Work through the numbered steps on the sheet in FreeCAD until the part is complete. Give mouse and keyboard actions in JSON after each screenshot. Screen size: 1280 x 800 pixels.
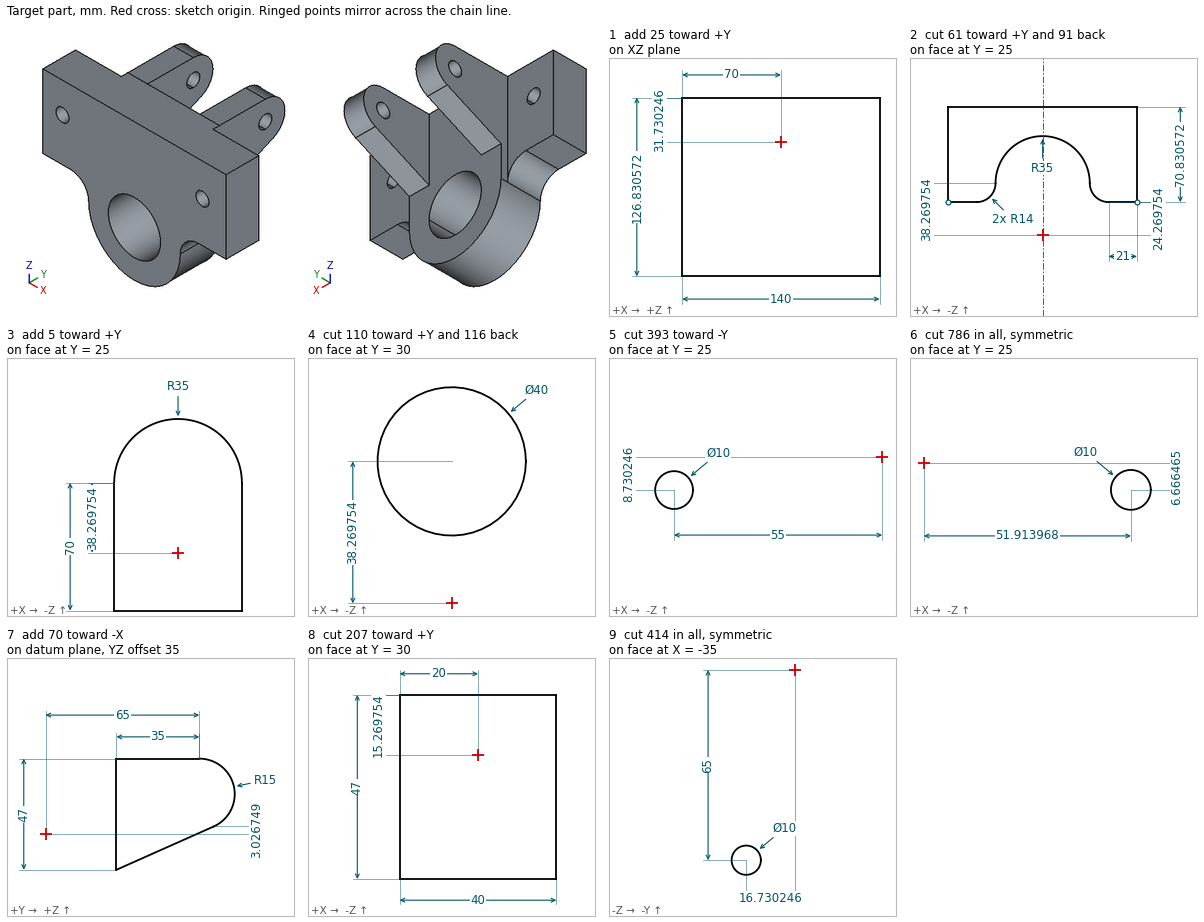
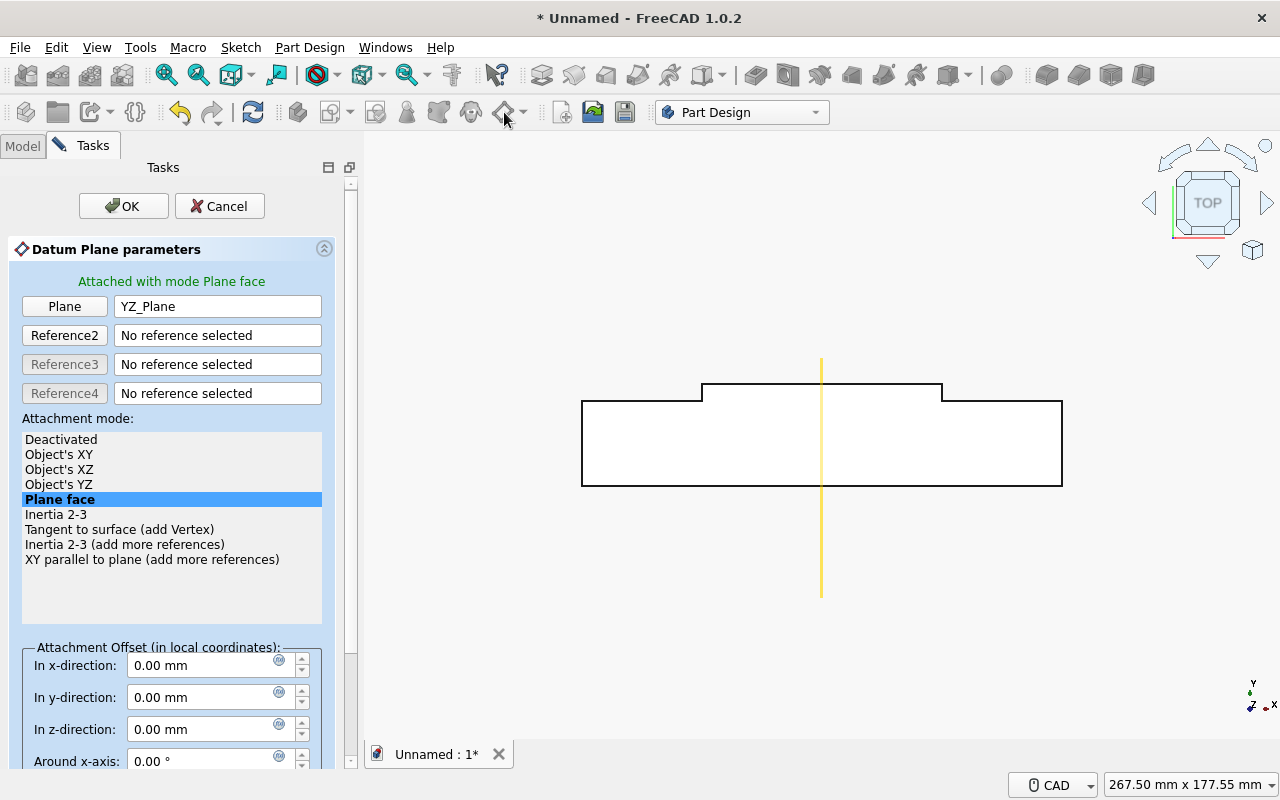
{"action": "triple_click", "coordinate": [210, 729]}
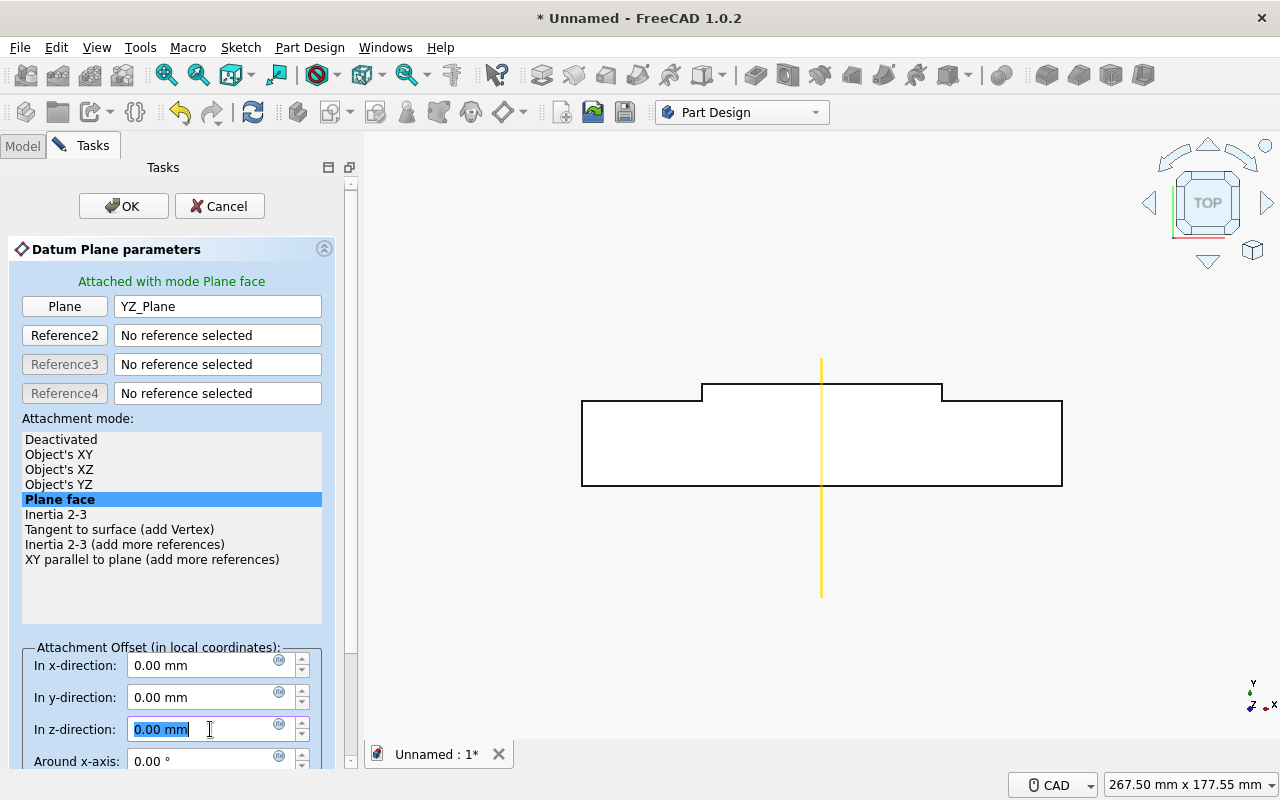
{"action": "type", "text": "35"}
{"action": "key", "text": "Tab"}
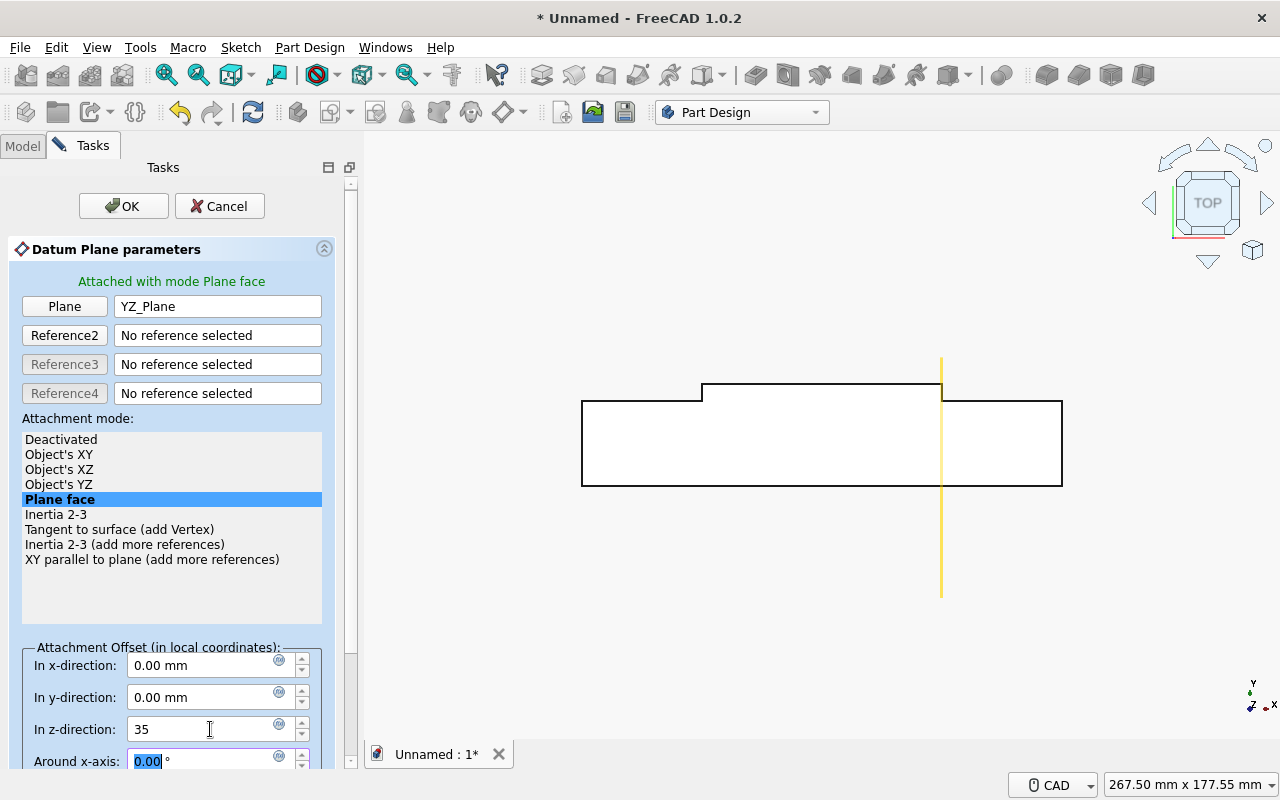
{"action": "left_click", "coordinate": [124, 206]}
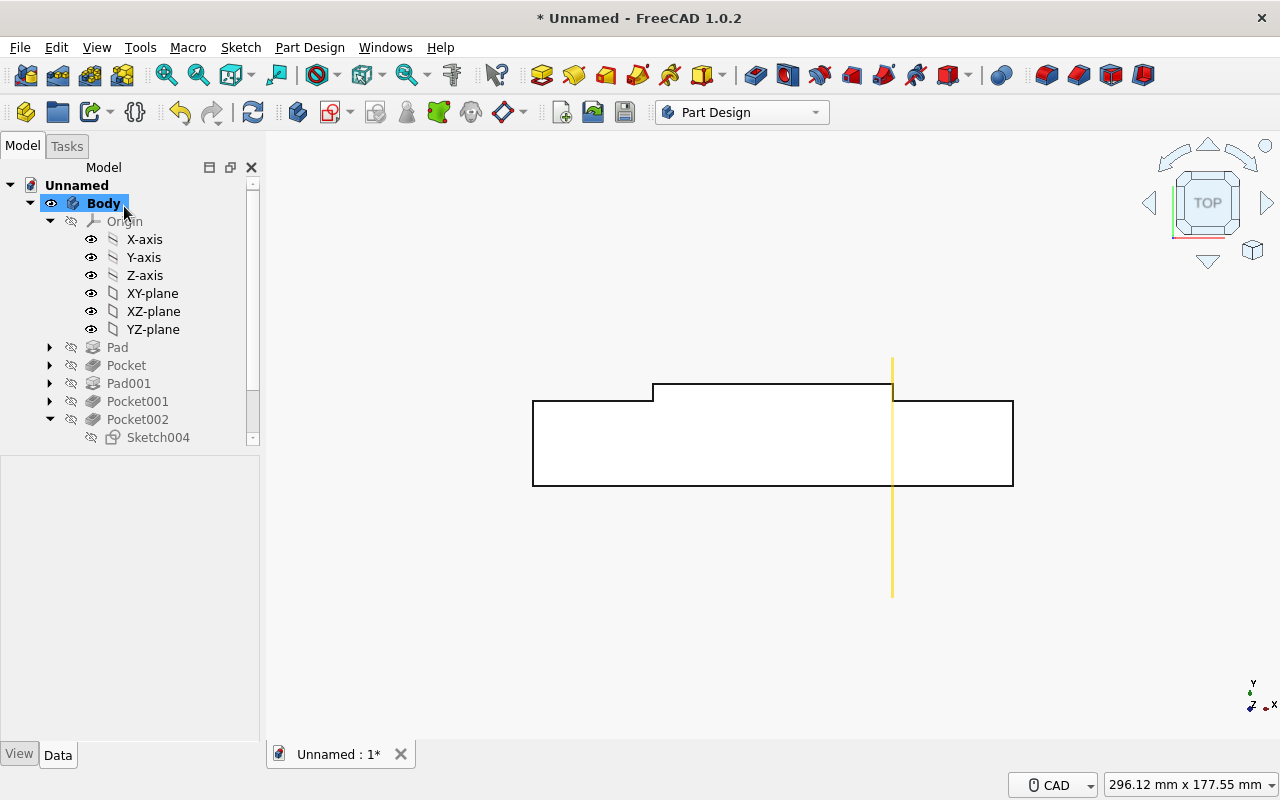
{"action": "scroll", "coordinate": [100, 307], "scroll_direction": "down", "scroll_amount": 3}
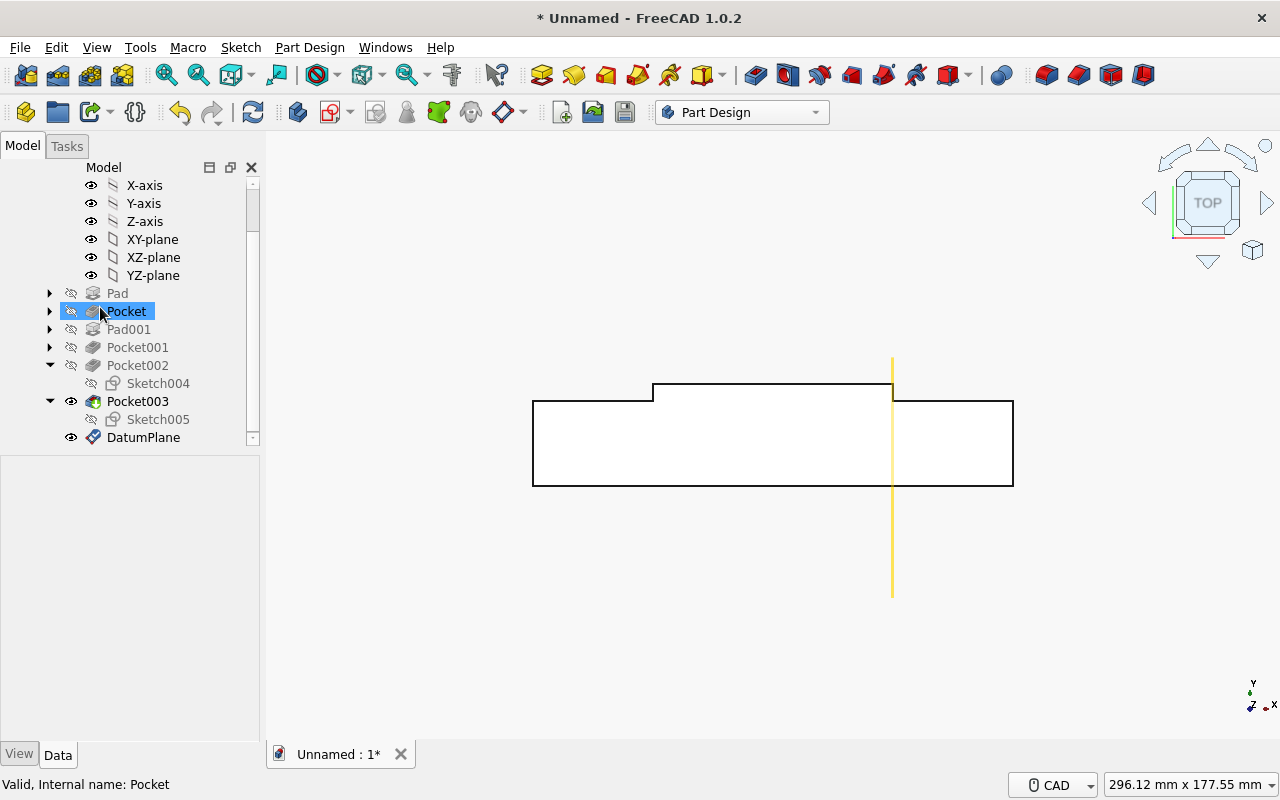
{"action": "left_click", "coordinate": [116, 437]}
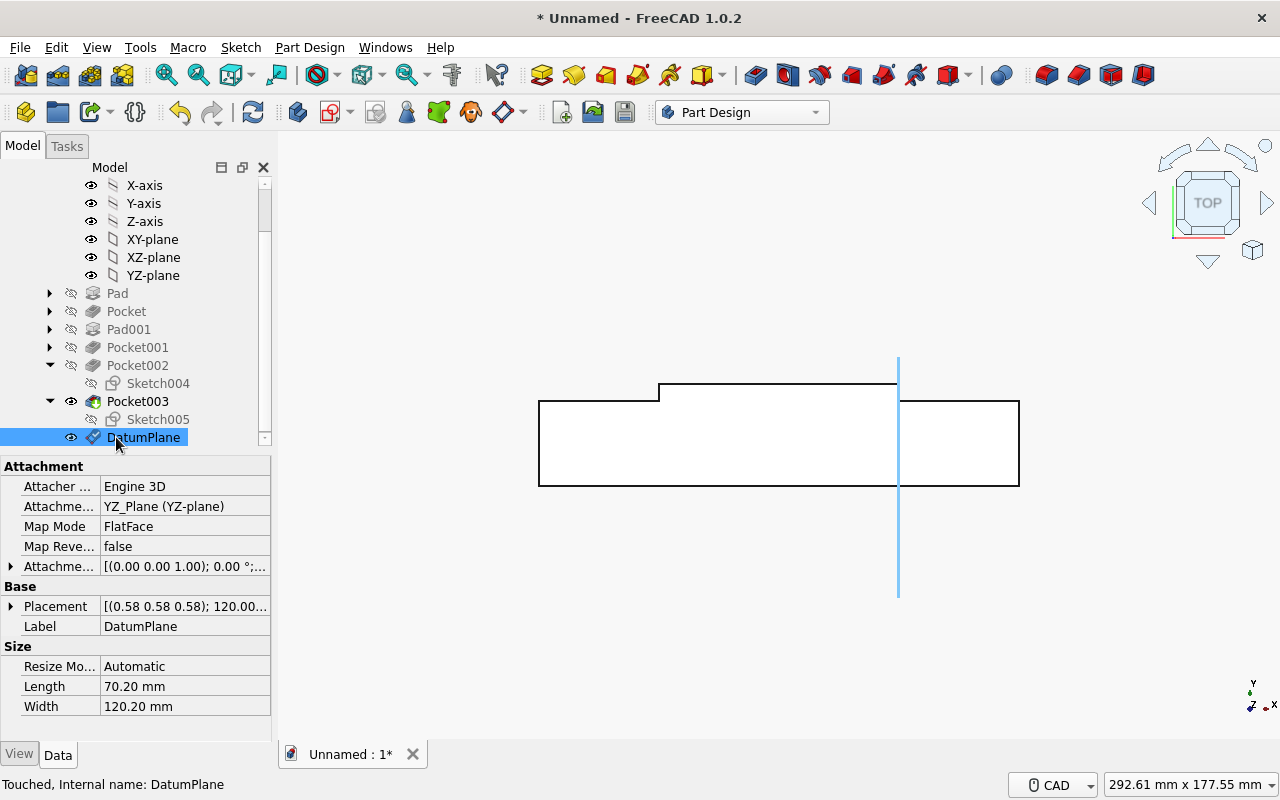
{"action": "left_click", "coordinate": [330, 112]}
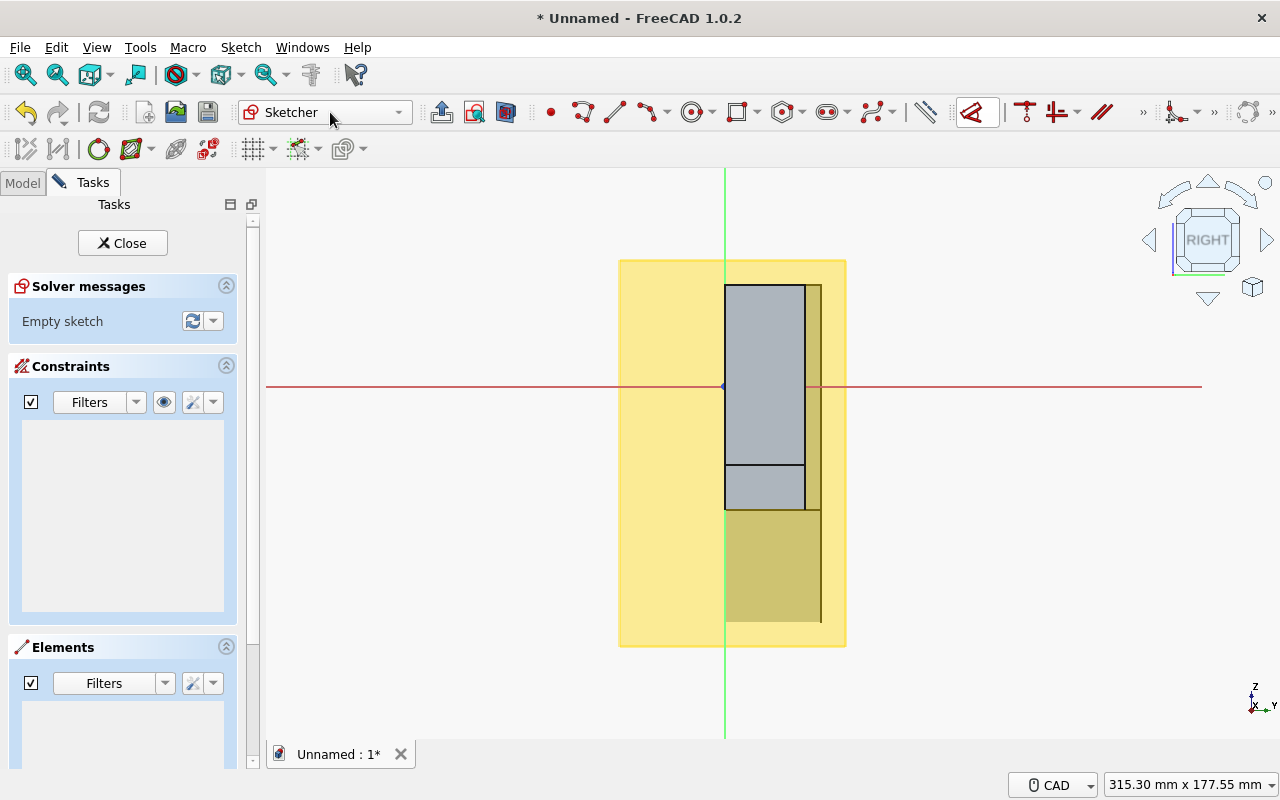
{"action": "left_click", "coordinate": [506, 112]}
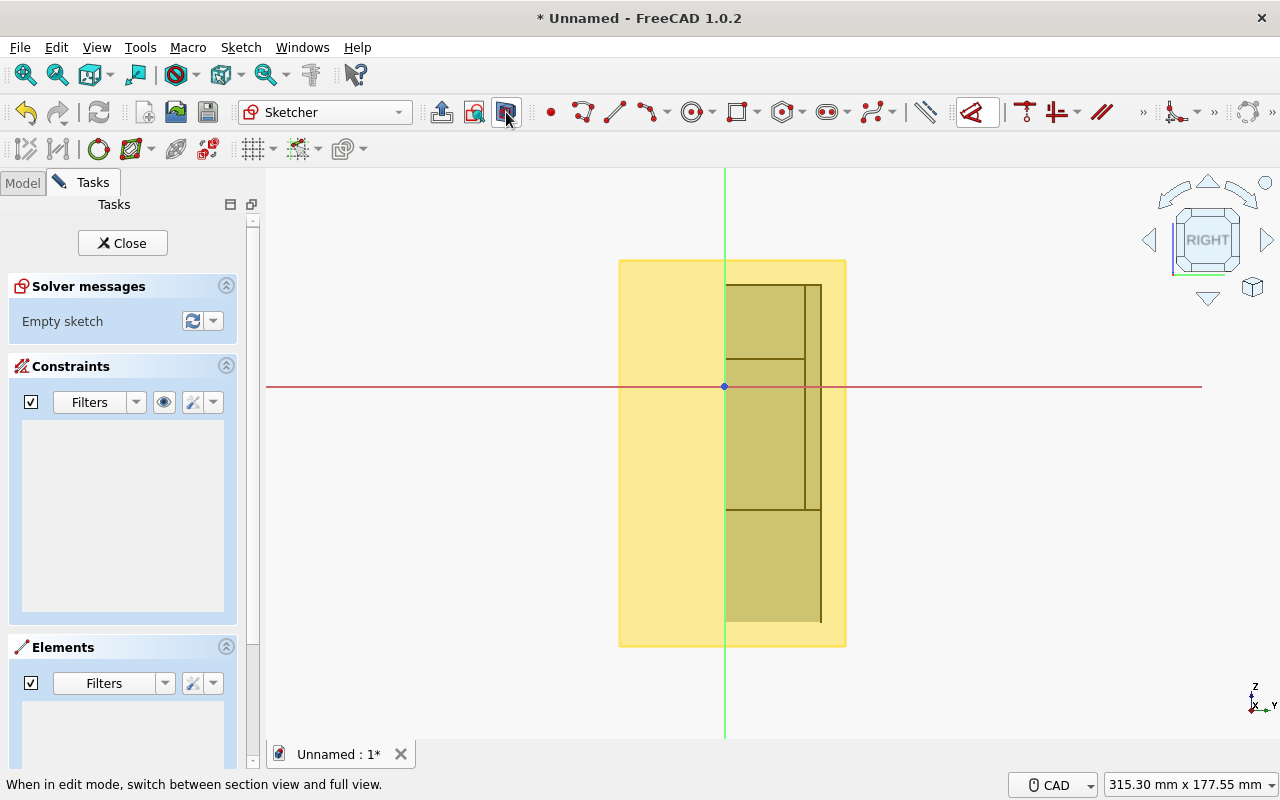
{"action": "scroll", "coordinate": [974, 284], "scroll_direction": "up", "scroll_amount": 4}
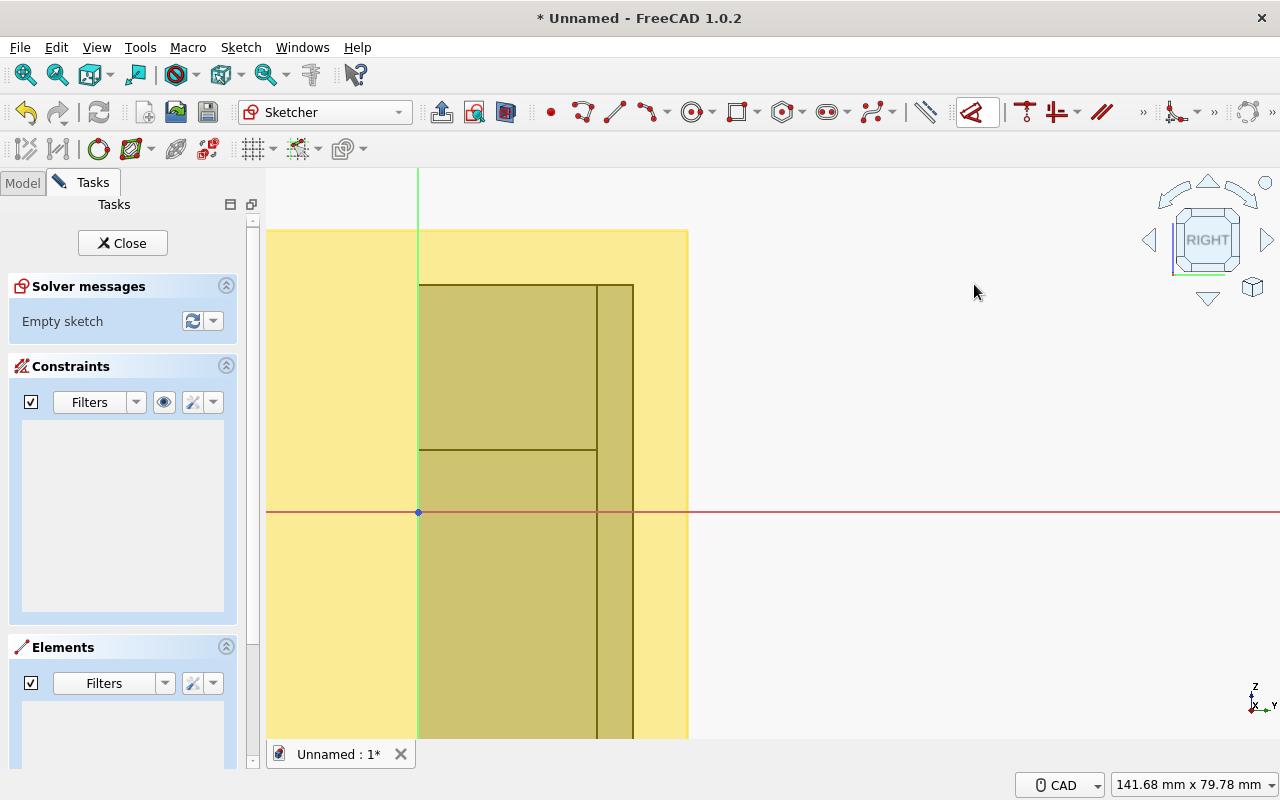
{"action": "left_click", "coordinate": [584, 112]}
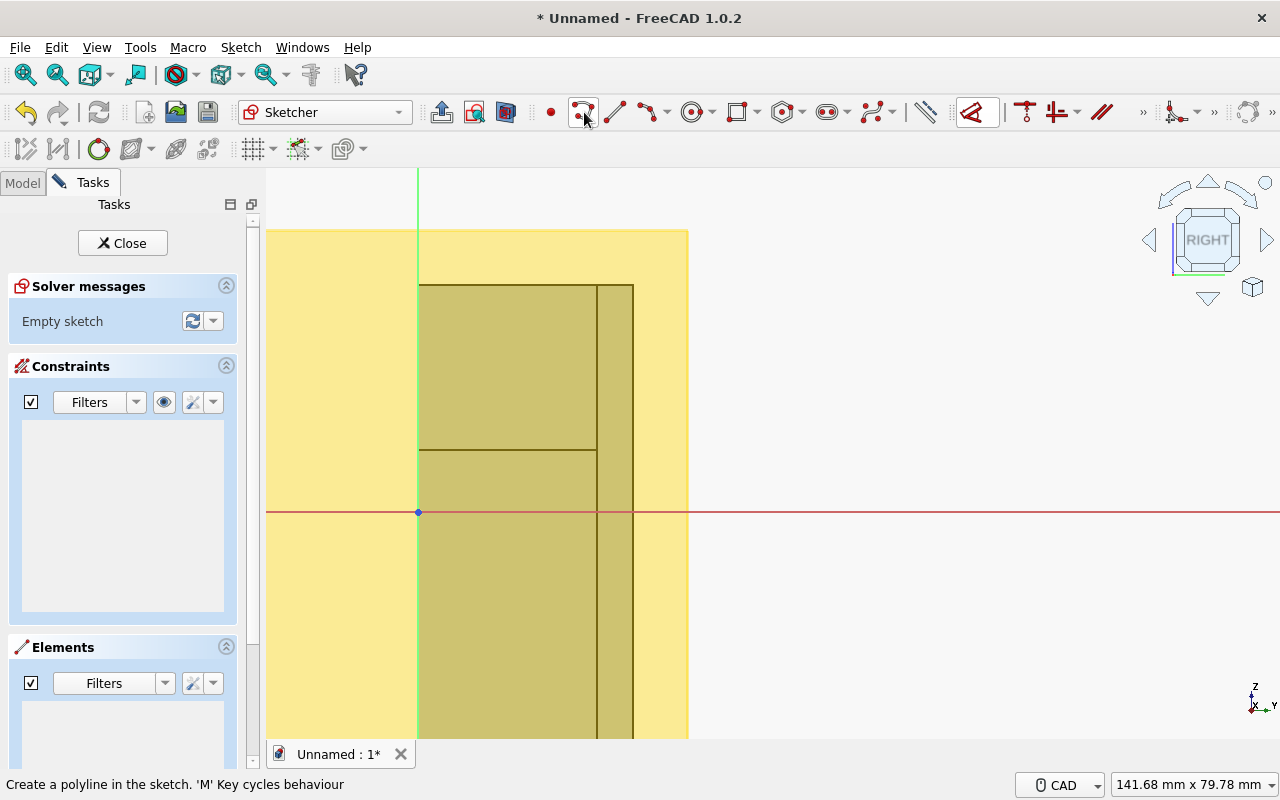
{"action": "left_click", "coordinate": [884, 285]}
{"action": "left_click", "coordinate": [633, 285]}
{"action": "left_click", "coordinate": [633, 622]}
{"action": "left_click", "coordinate": [927, 491]}
{"action": "right_click", "coordinate": [927, 491]}